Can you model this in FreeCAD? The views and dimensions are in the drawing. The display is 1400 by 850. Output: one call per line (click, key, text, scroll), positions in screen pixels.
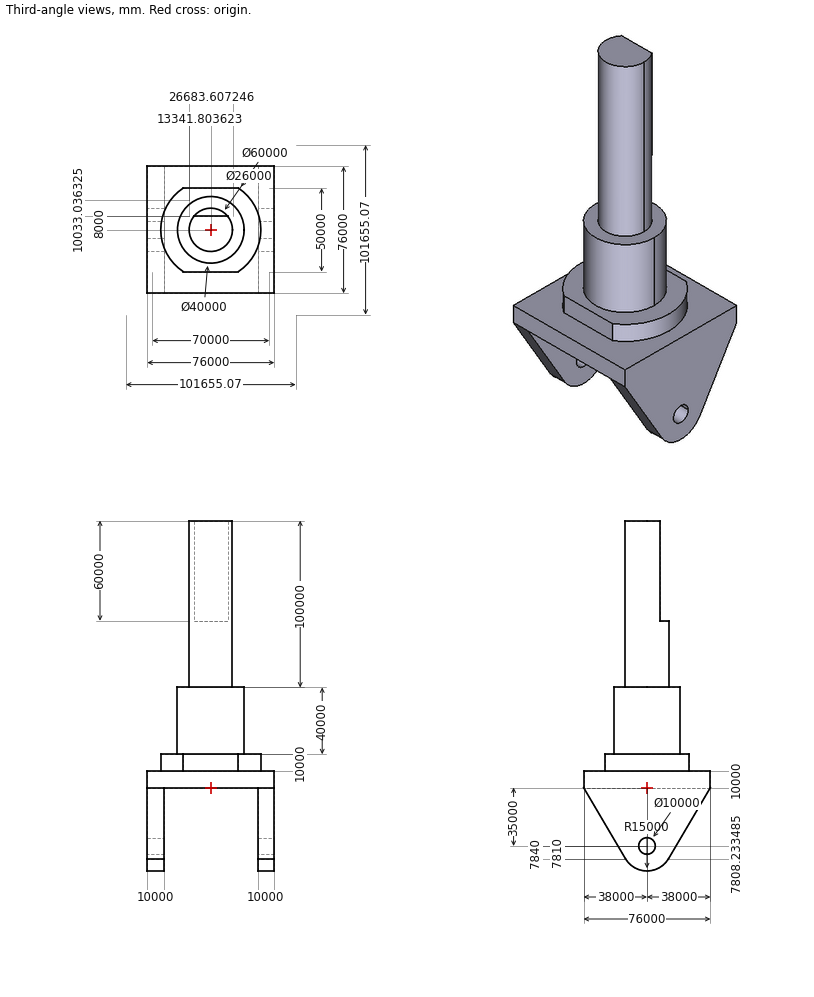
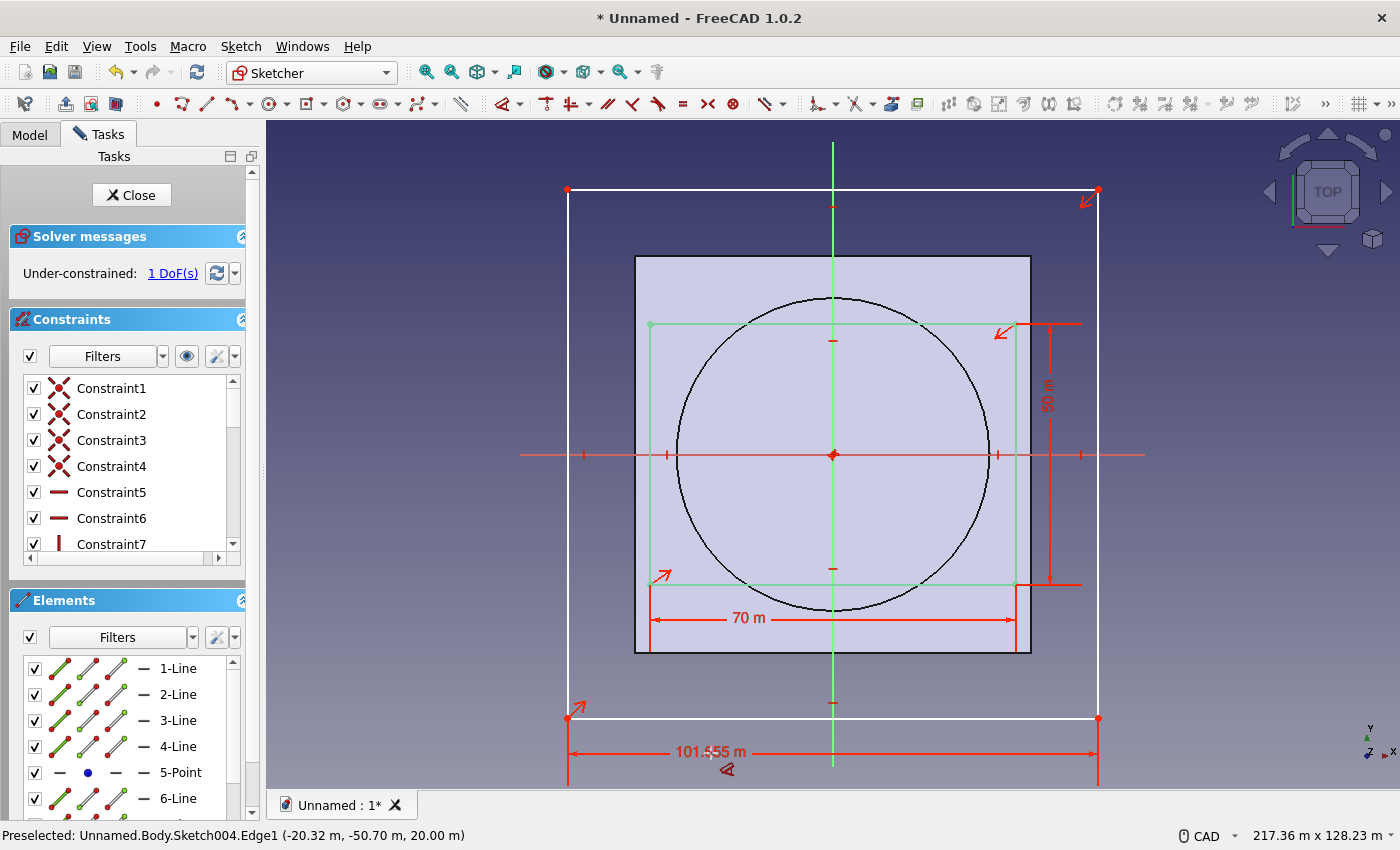
click(1098, 560)
click(1132, 333)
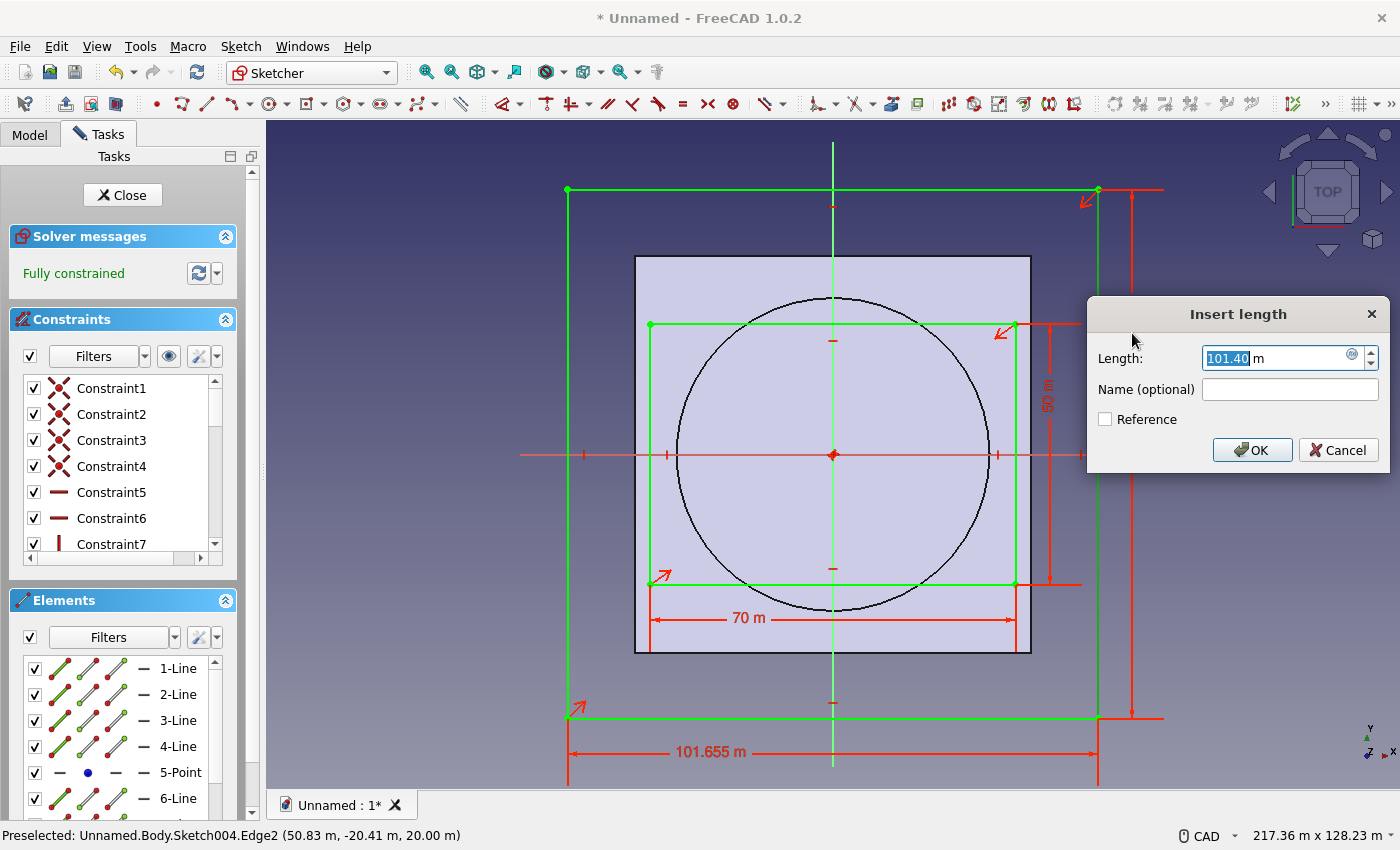
key(ctrl+a)
text(101655.07 mm)
key(Return)
key(Escape)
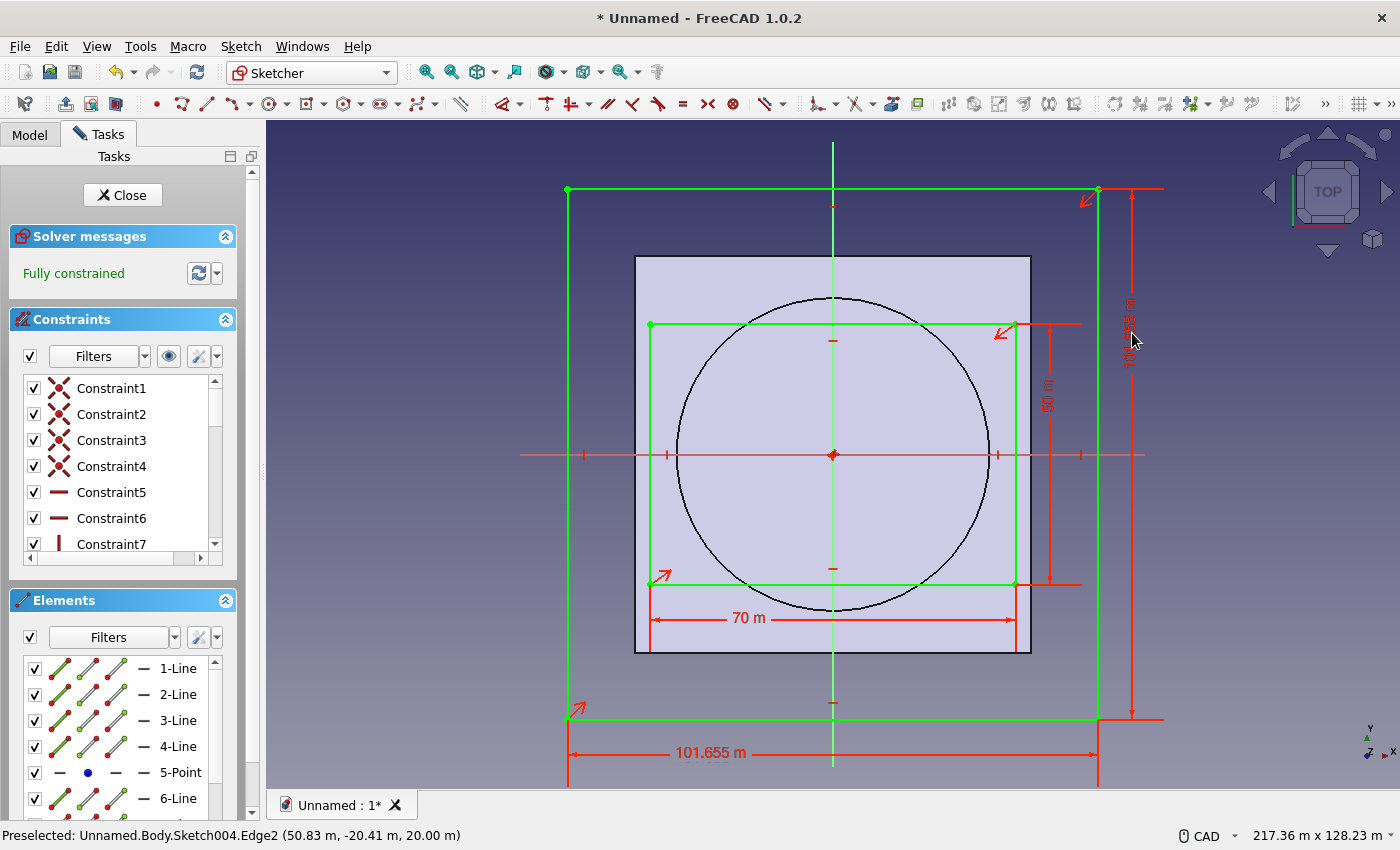
click(123, 195)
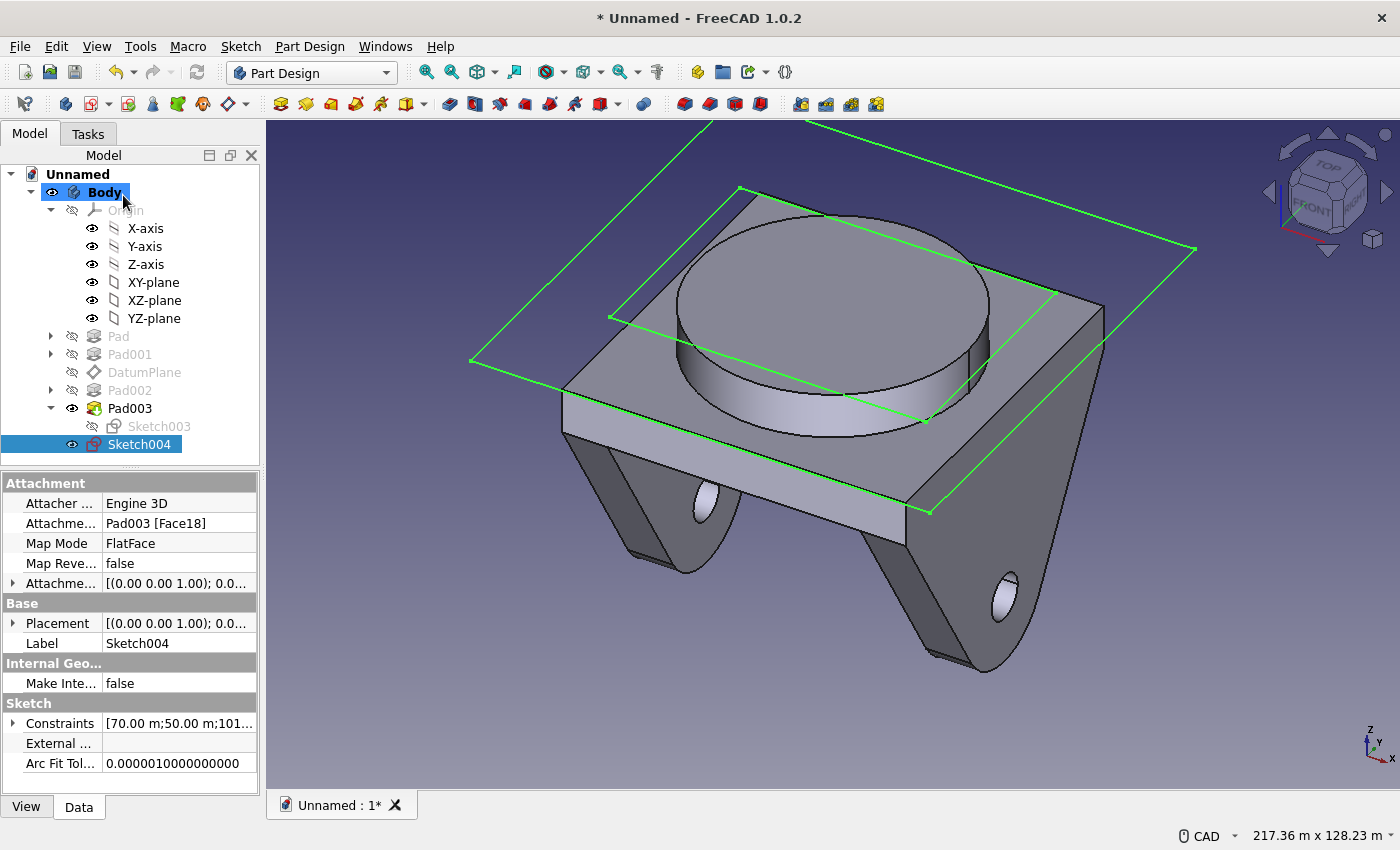
click(450, 104)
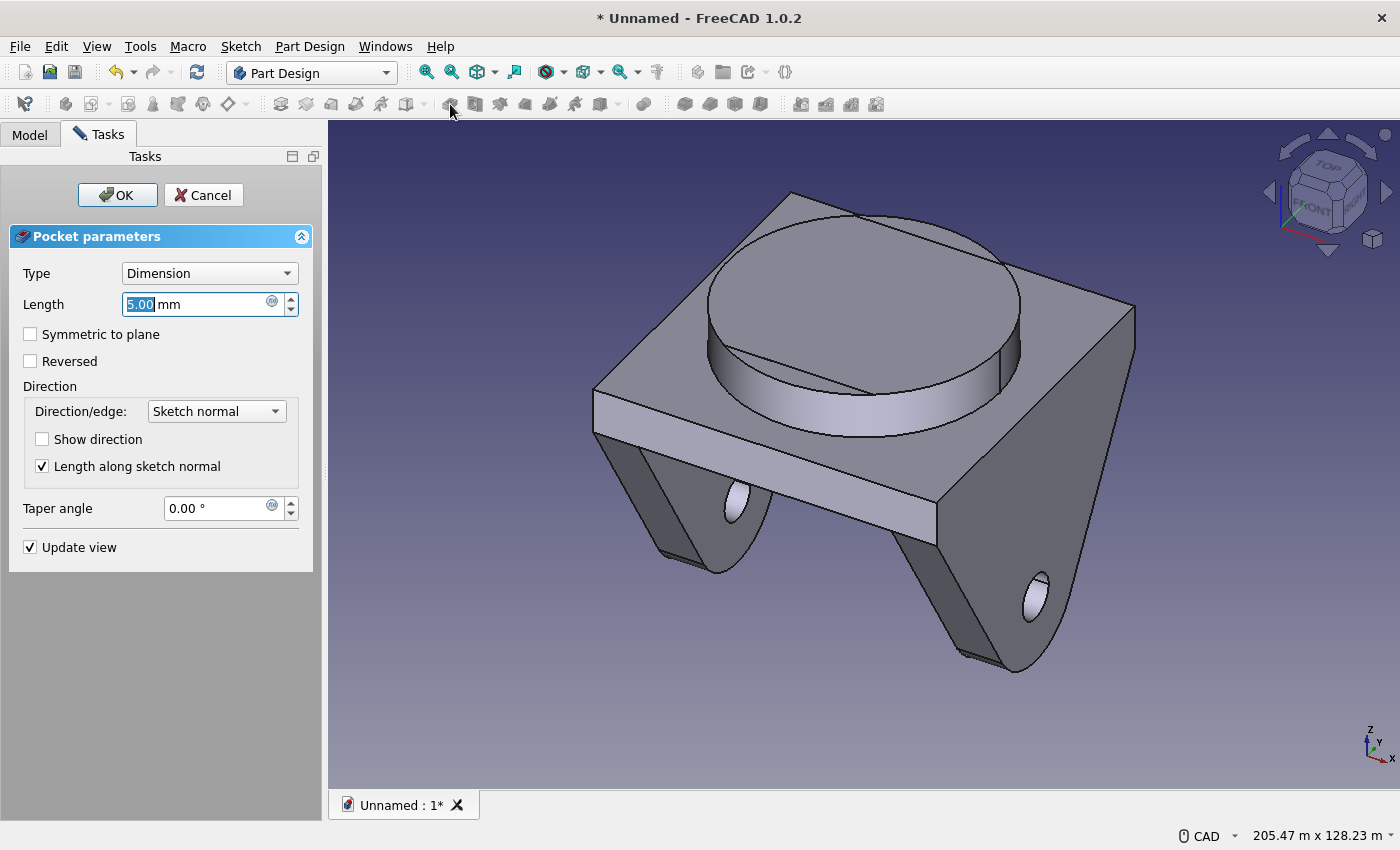
text(10000)
key(Tab)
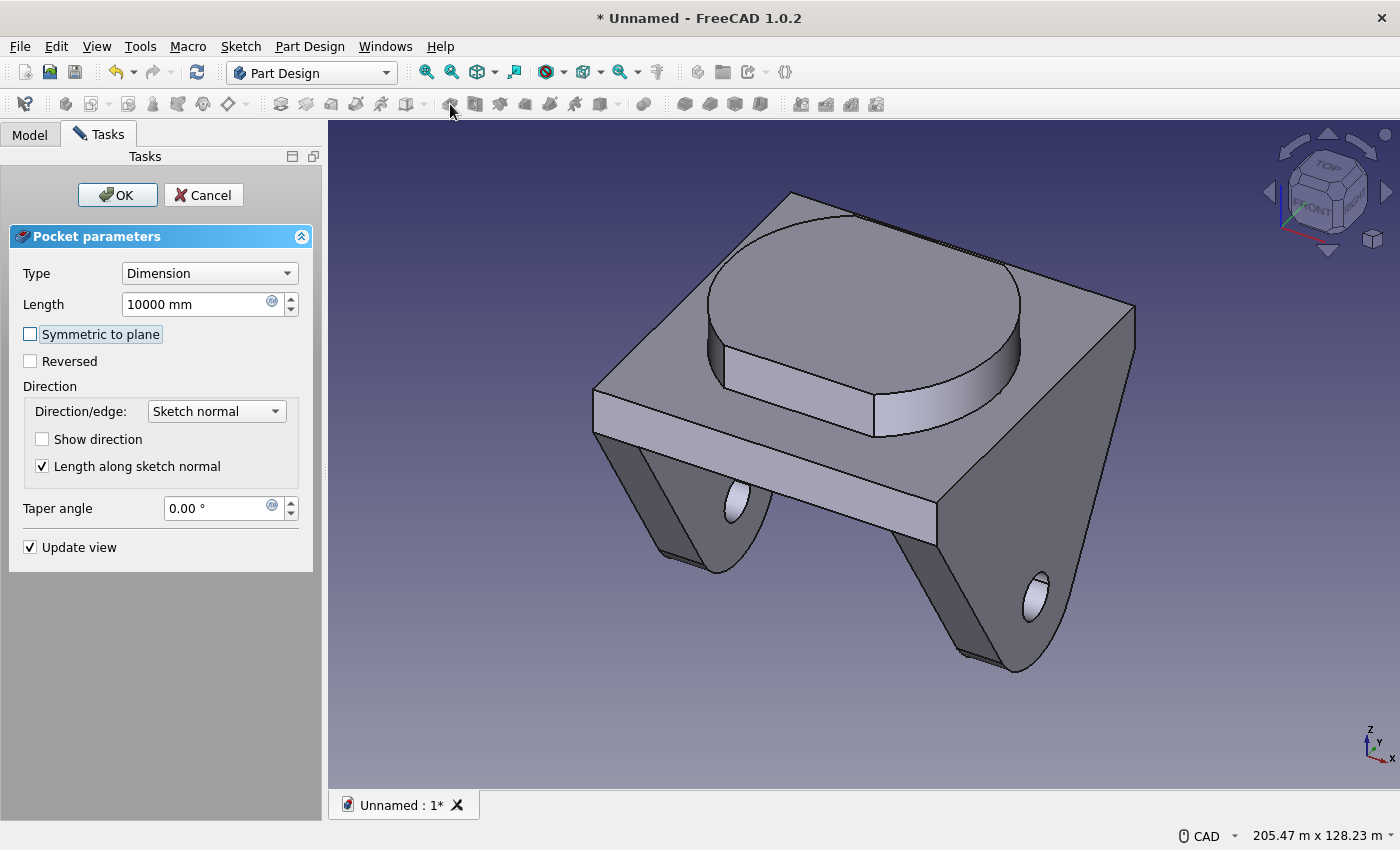
click(118, 195)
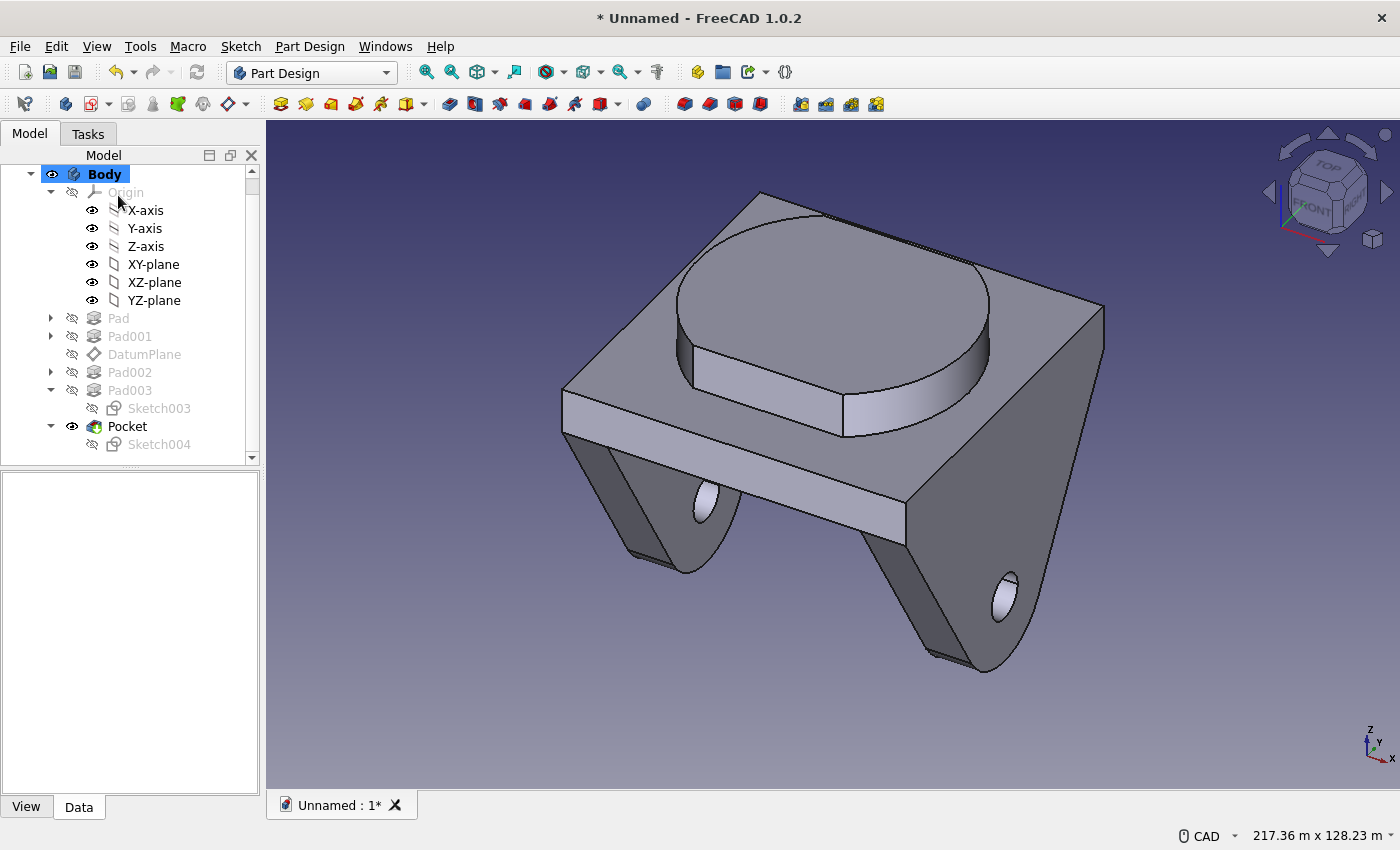
click(833, 304)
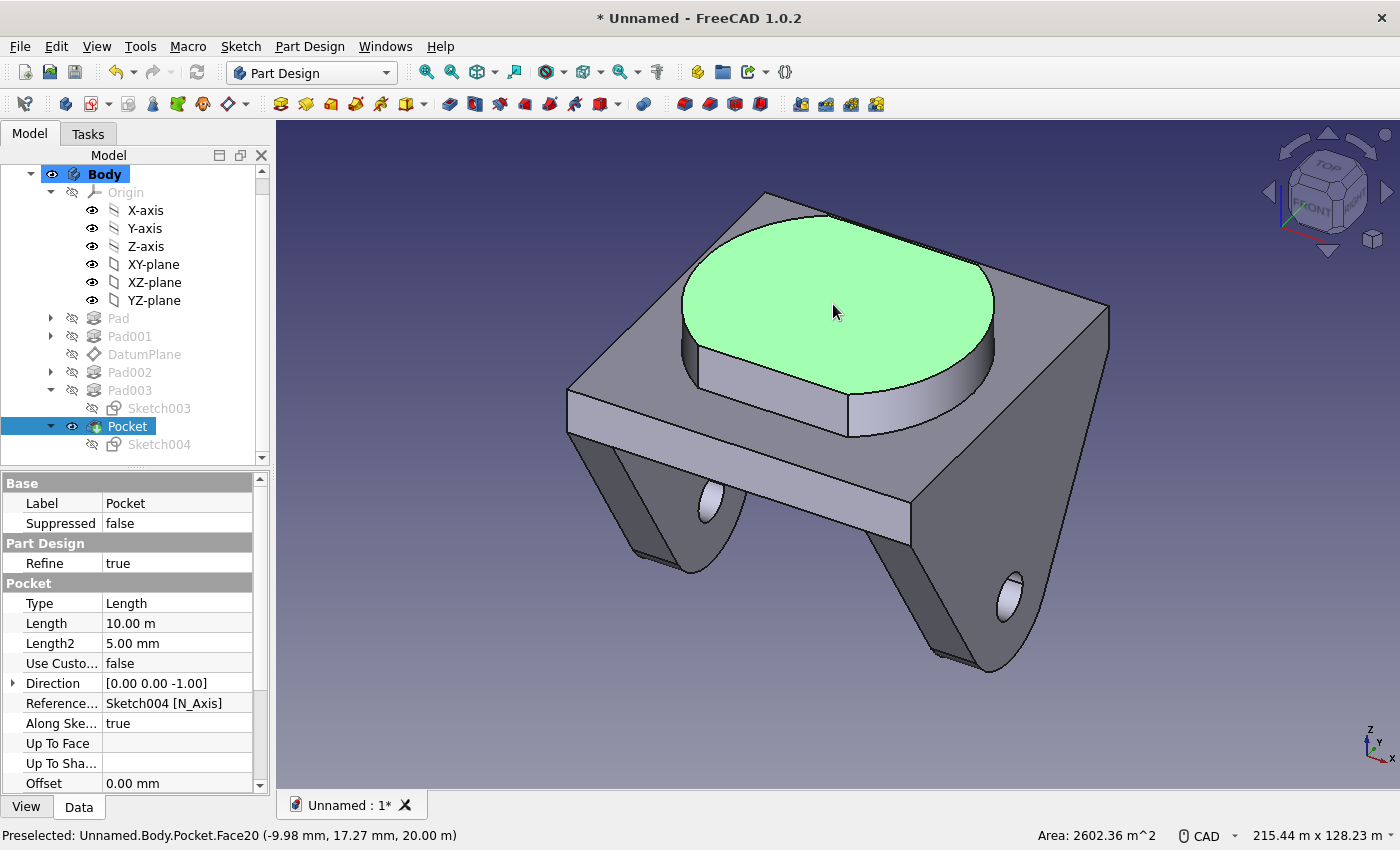
click(90, 104)